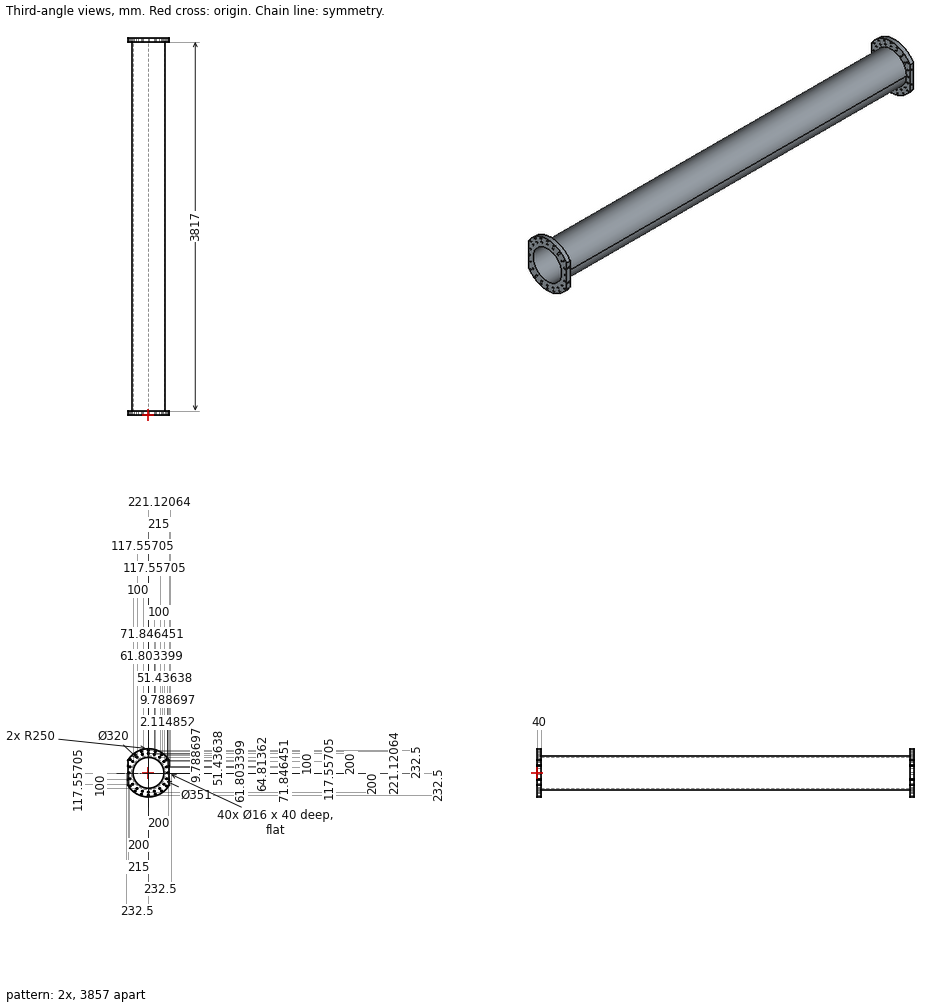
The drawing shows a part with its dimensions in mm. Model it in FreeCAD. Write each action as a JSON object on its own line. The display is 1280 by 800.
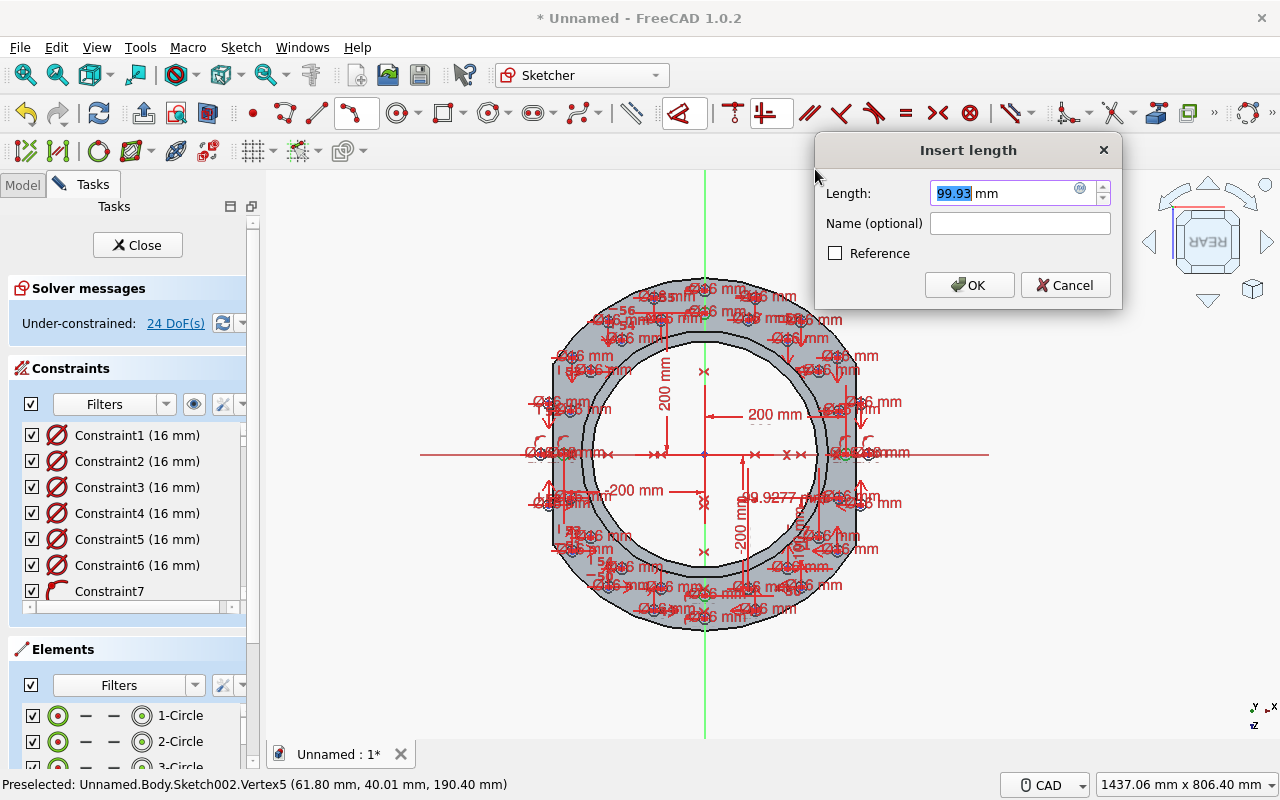
{"action": "type", "text": "100"}
{"action": "key", "text": "Return"}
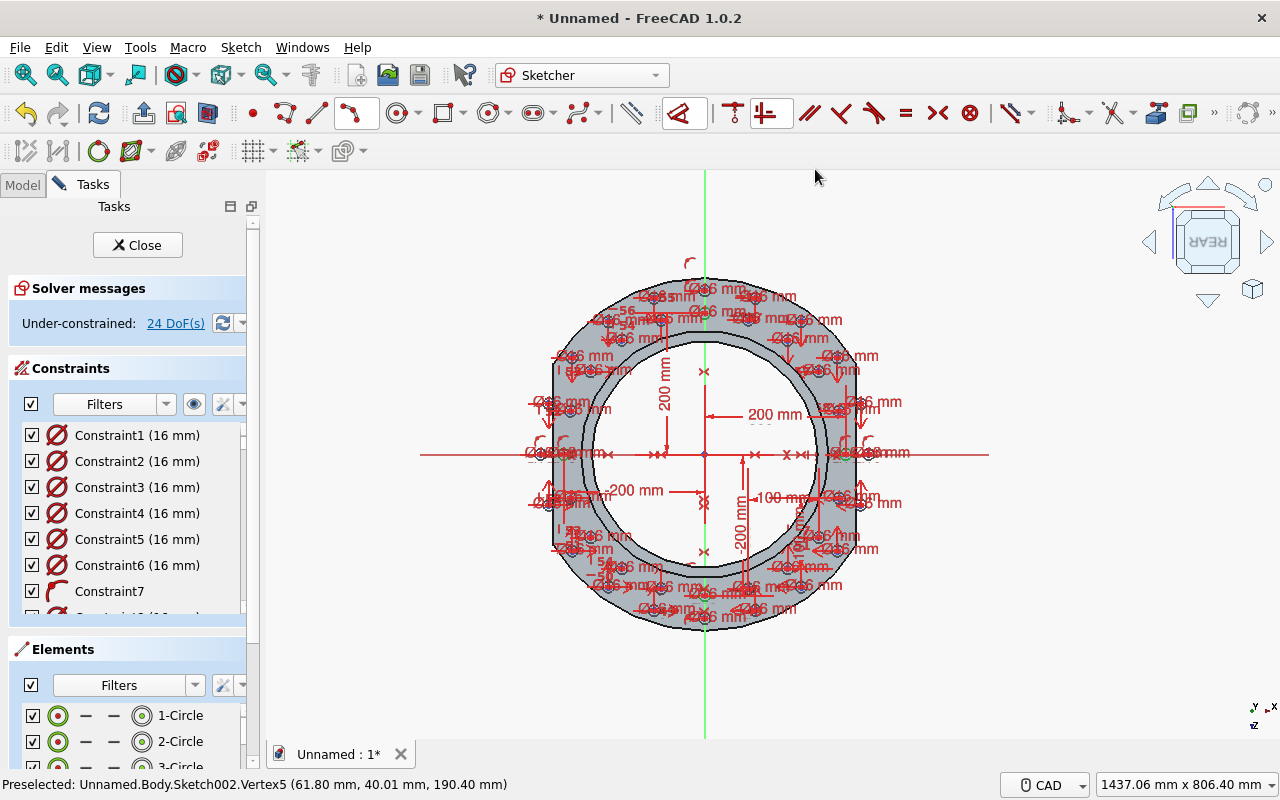
{"action": "left_click", "coordinate": [661, 589]}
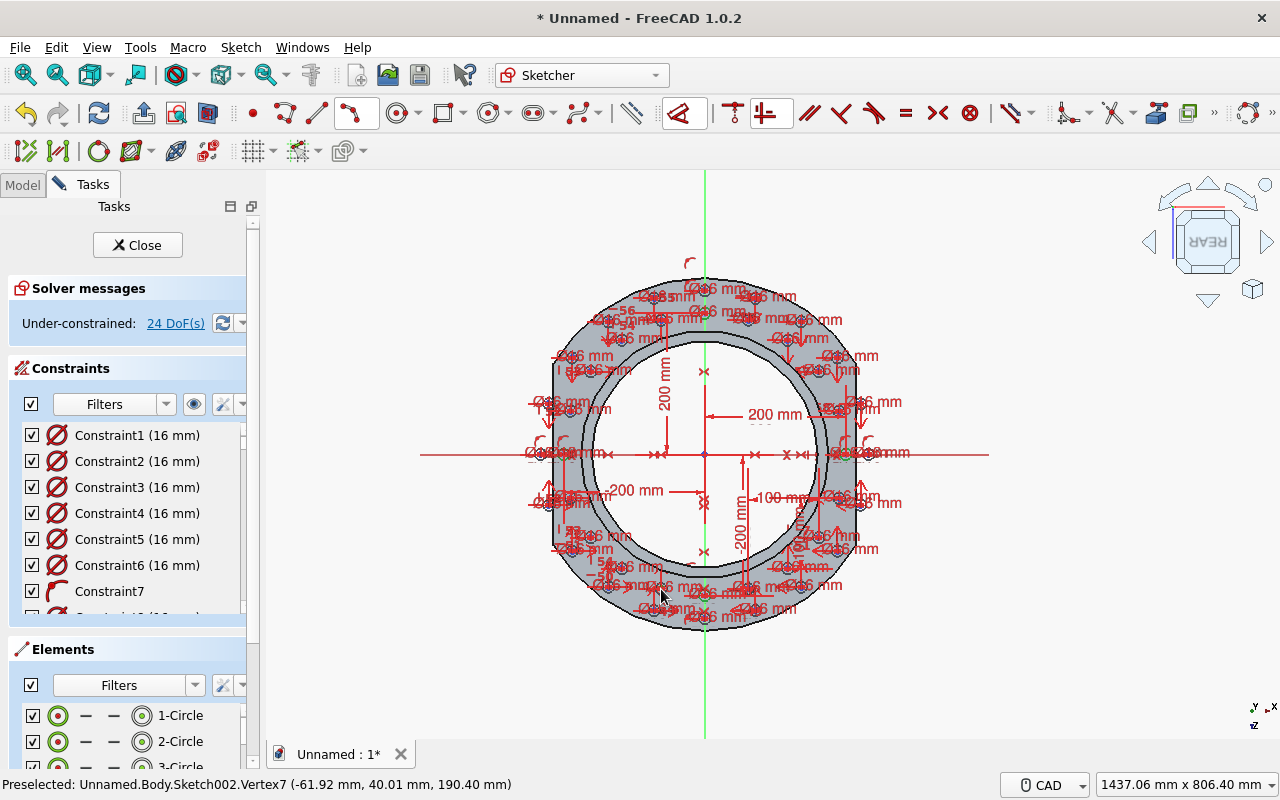
{"action": "left_click", "coordinate": [591, 538]}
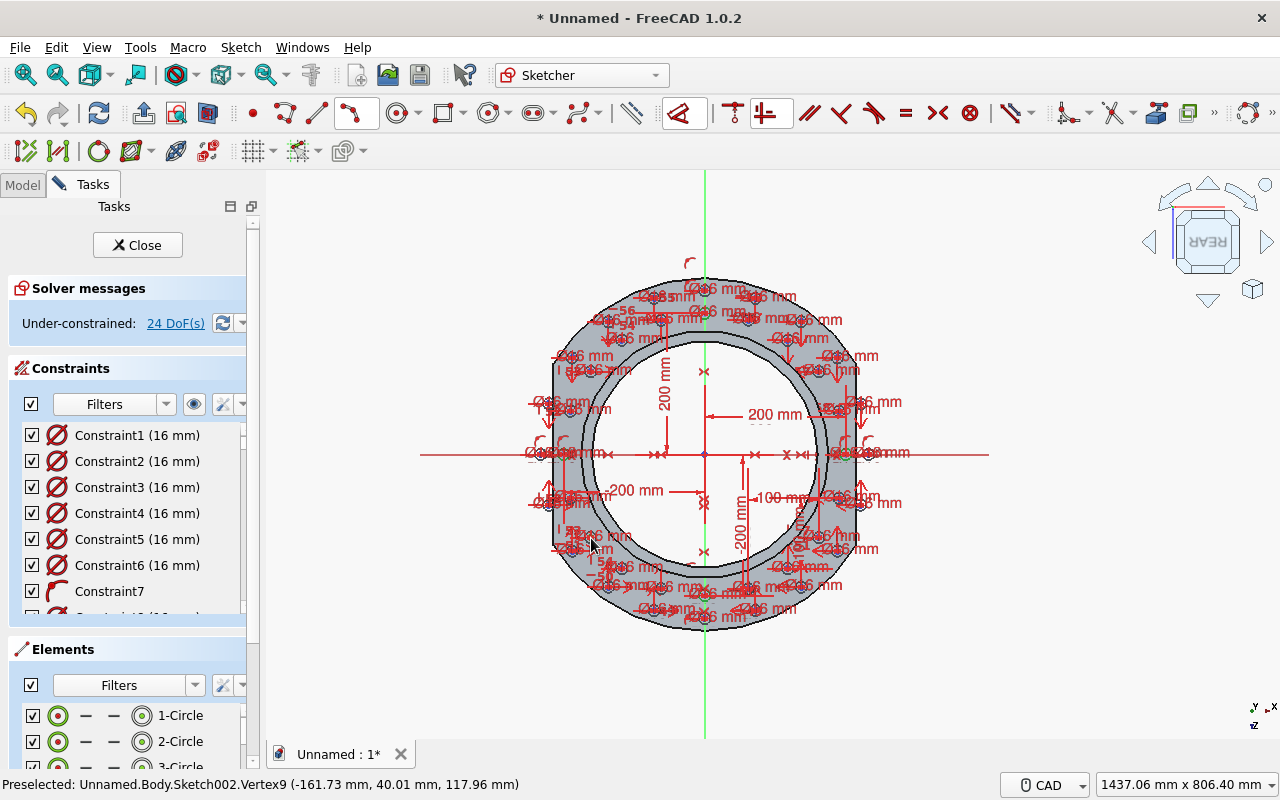
{"action": "key", "text": "l"}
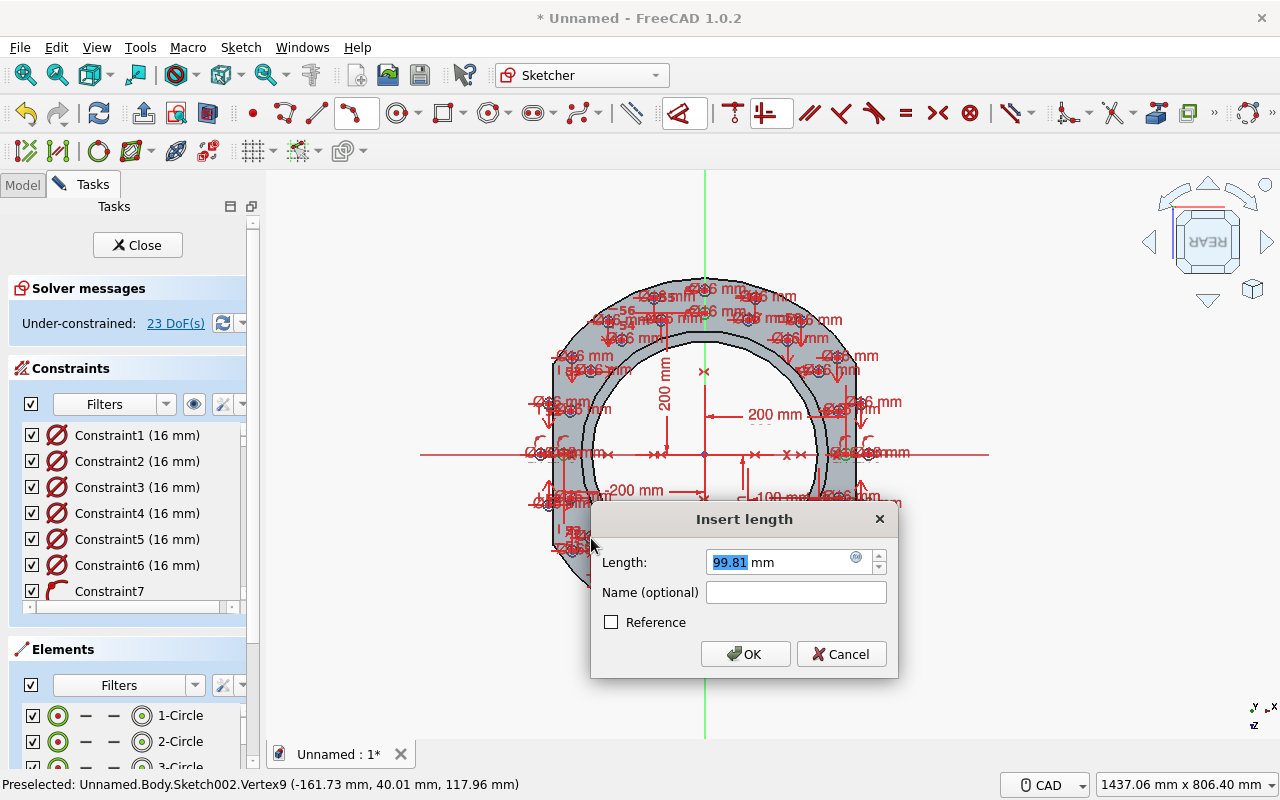
{"action": "type", "text": "100"}
{"action": "key", "text": "Return"}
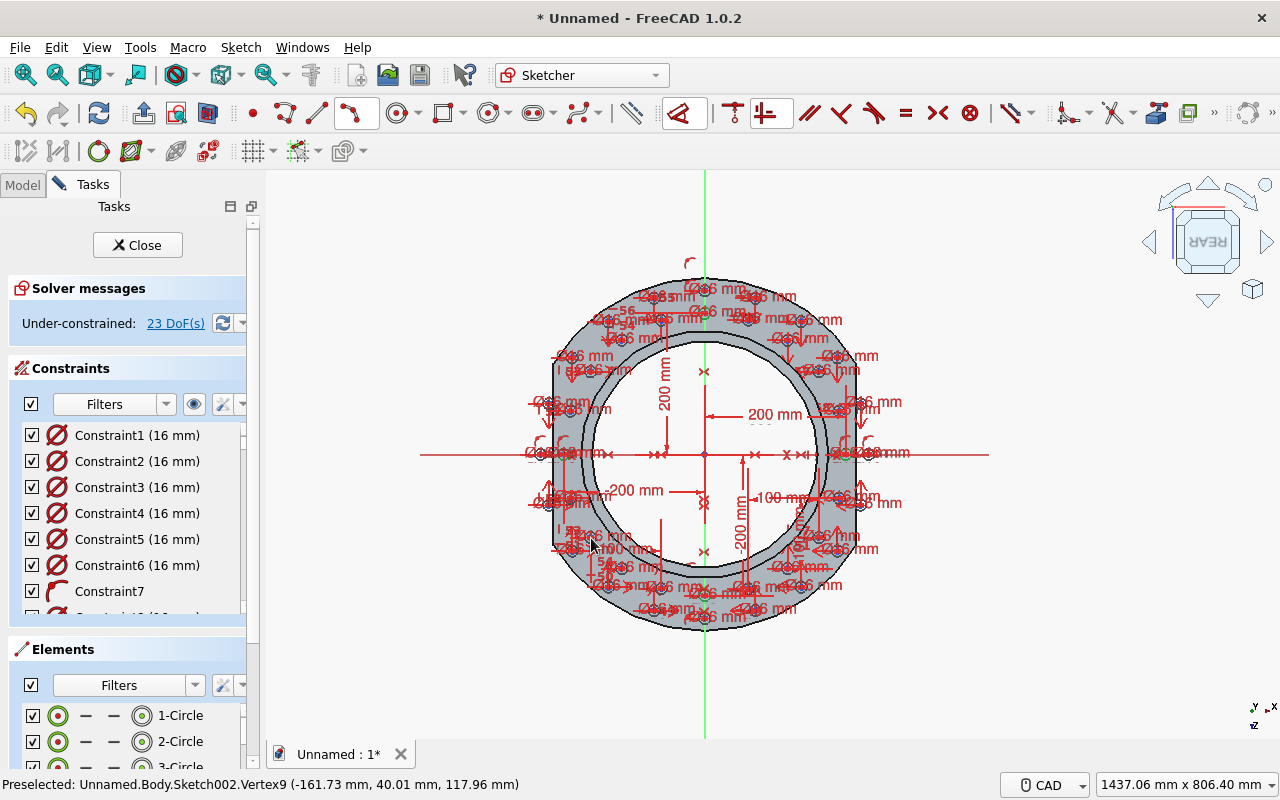
{"action": "left_click", "coordinate": [570, 411]}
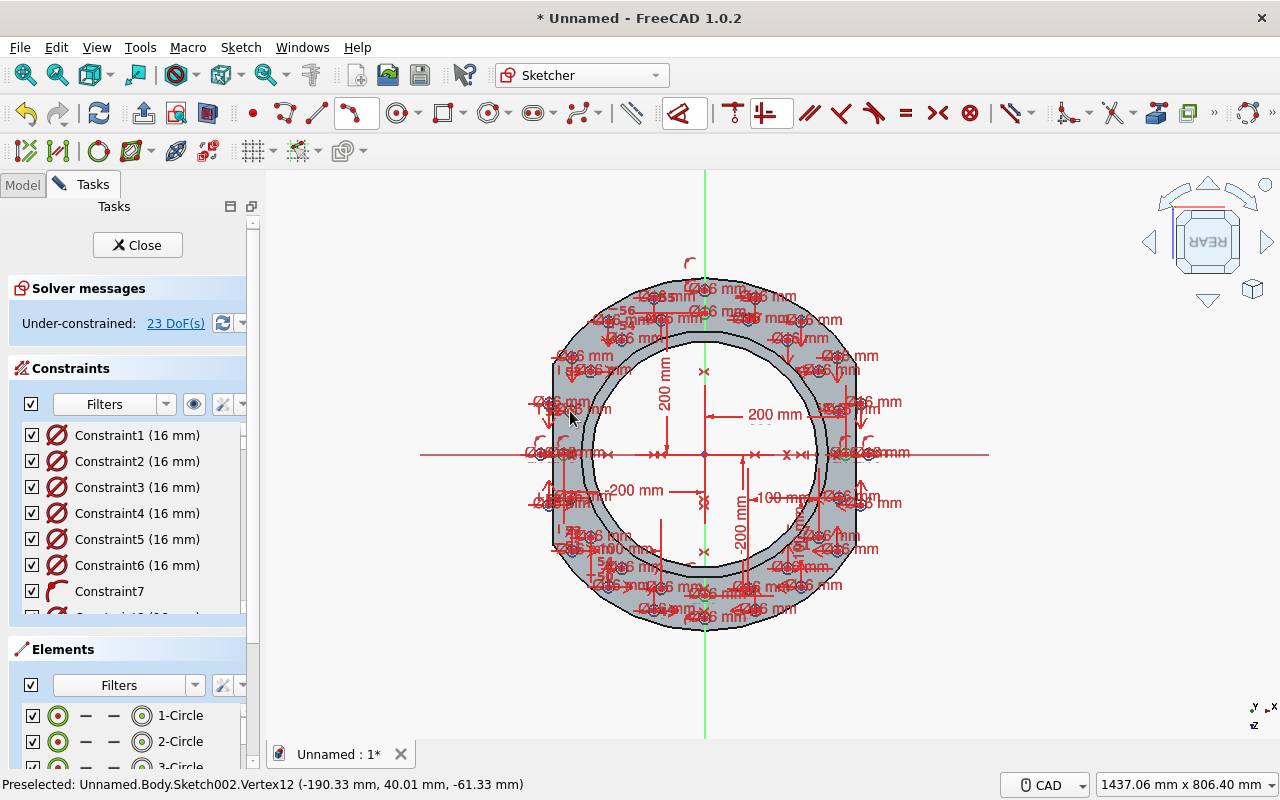
{"action": "left_click", "coordinate": [622, 340]}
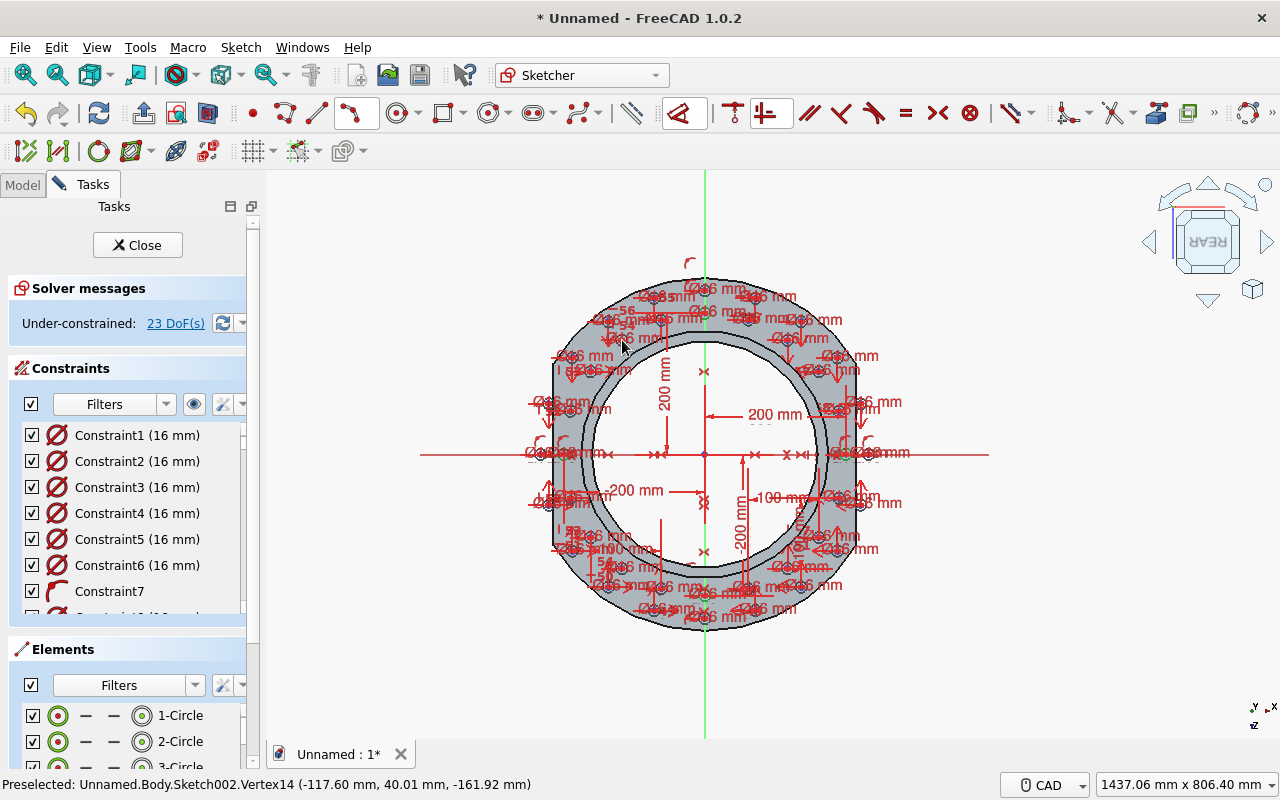
{"action": "left_click", "coordinate": [702, 114]}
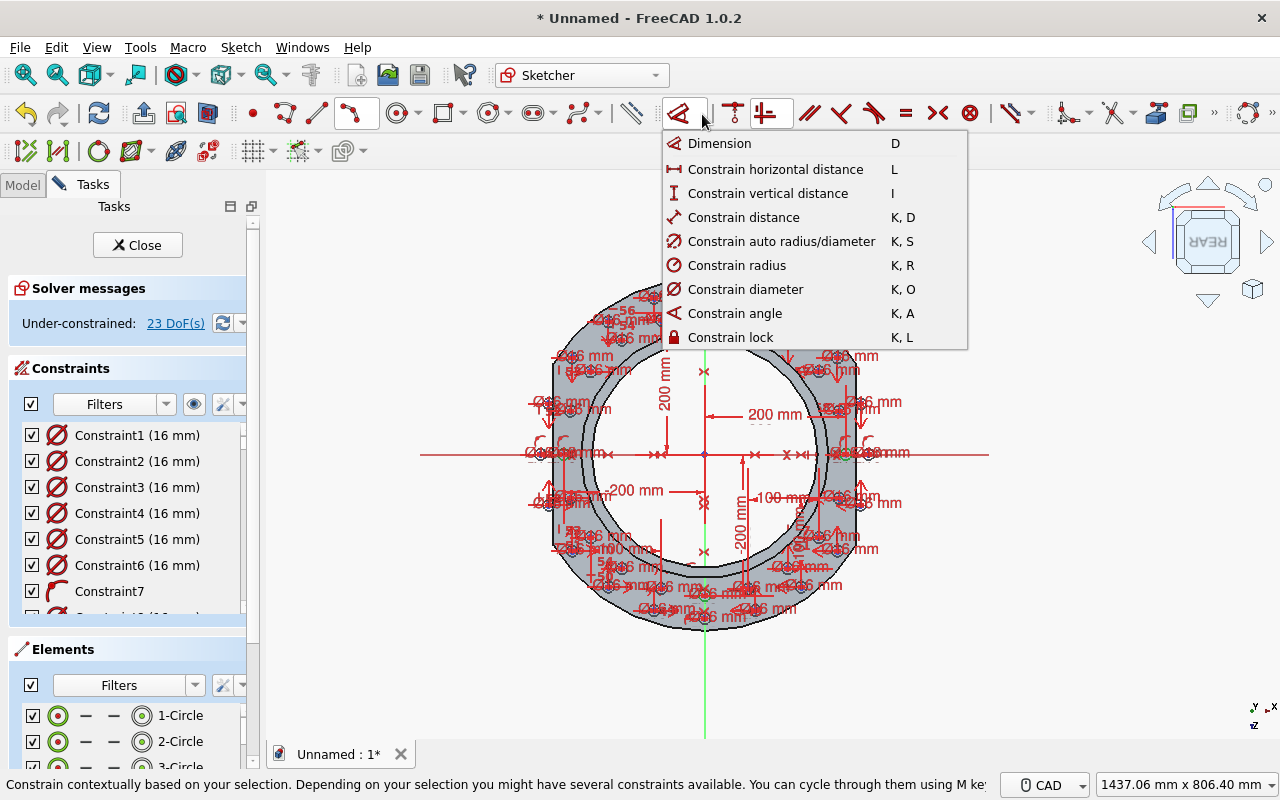
{"action": "left_click", "coordinate": [815, 193]}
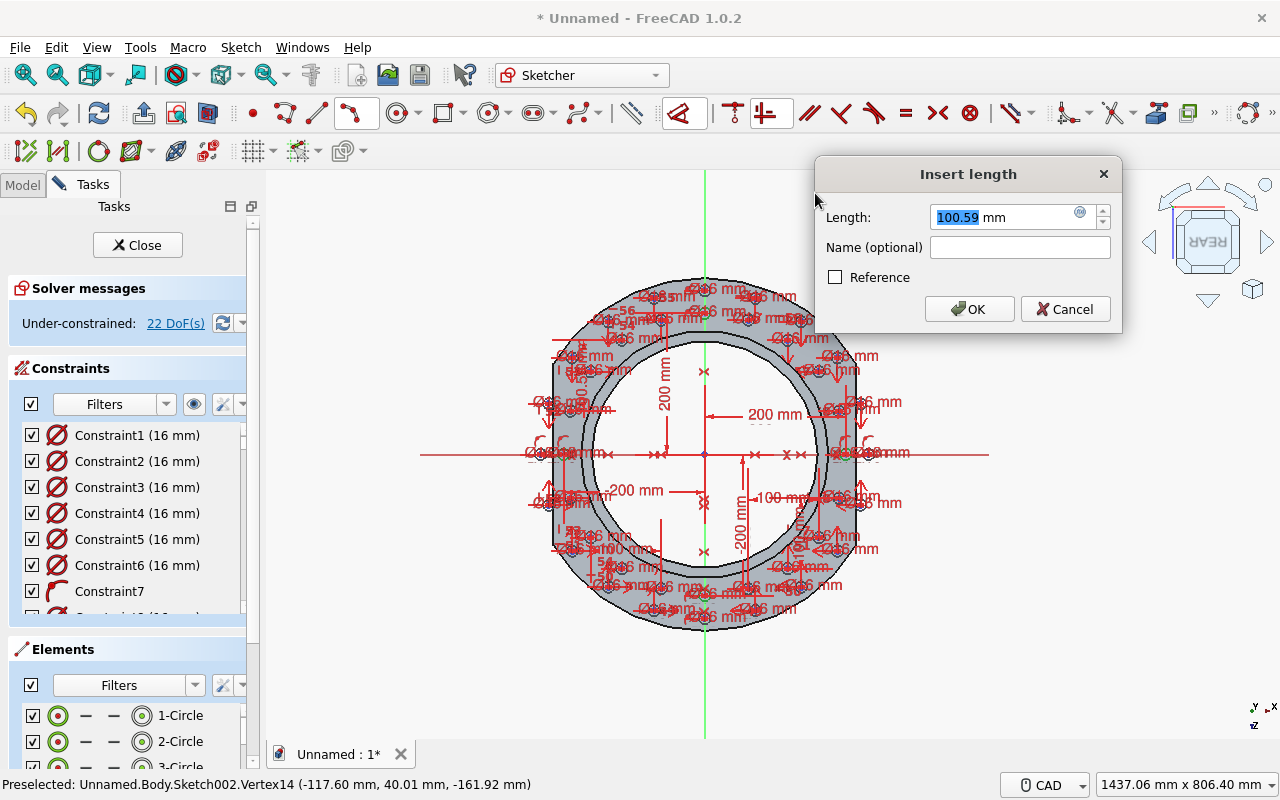
{"action": "type", "text": "100"}
{"action": "key", "text": "Return"}